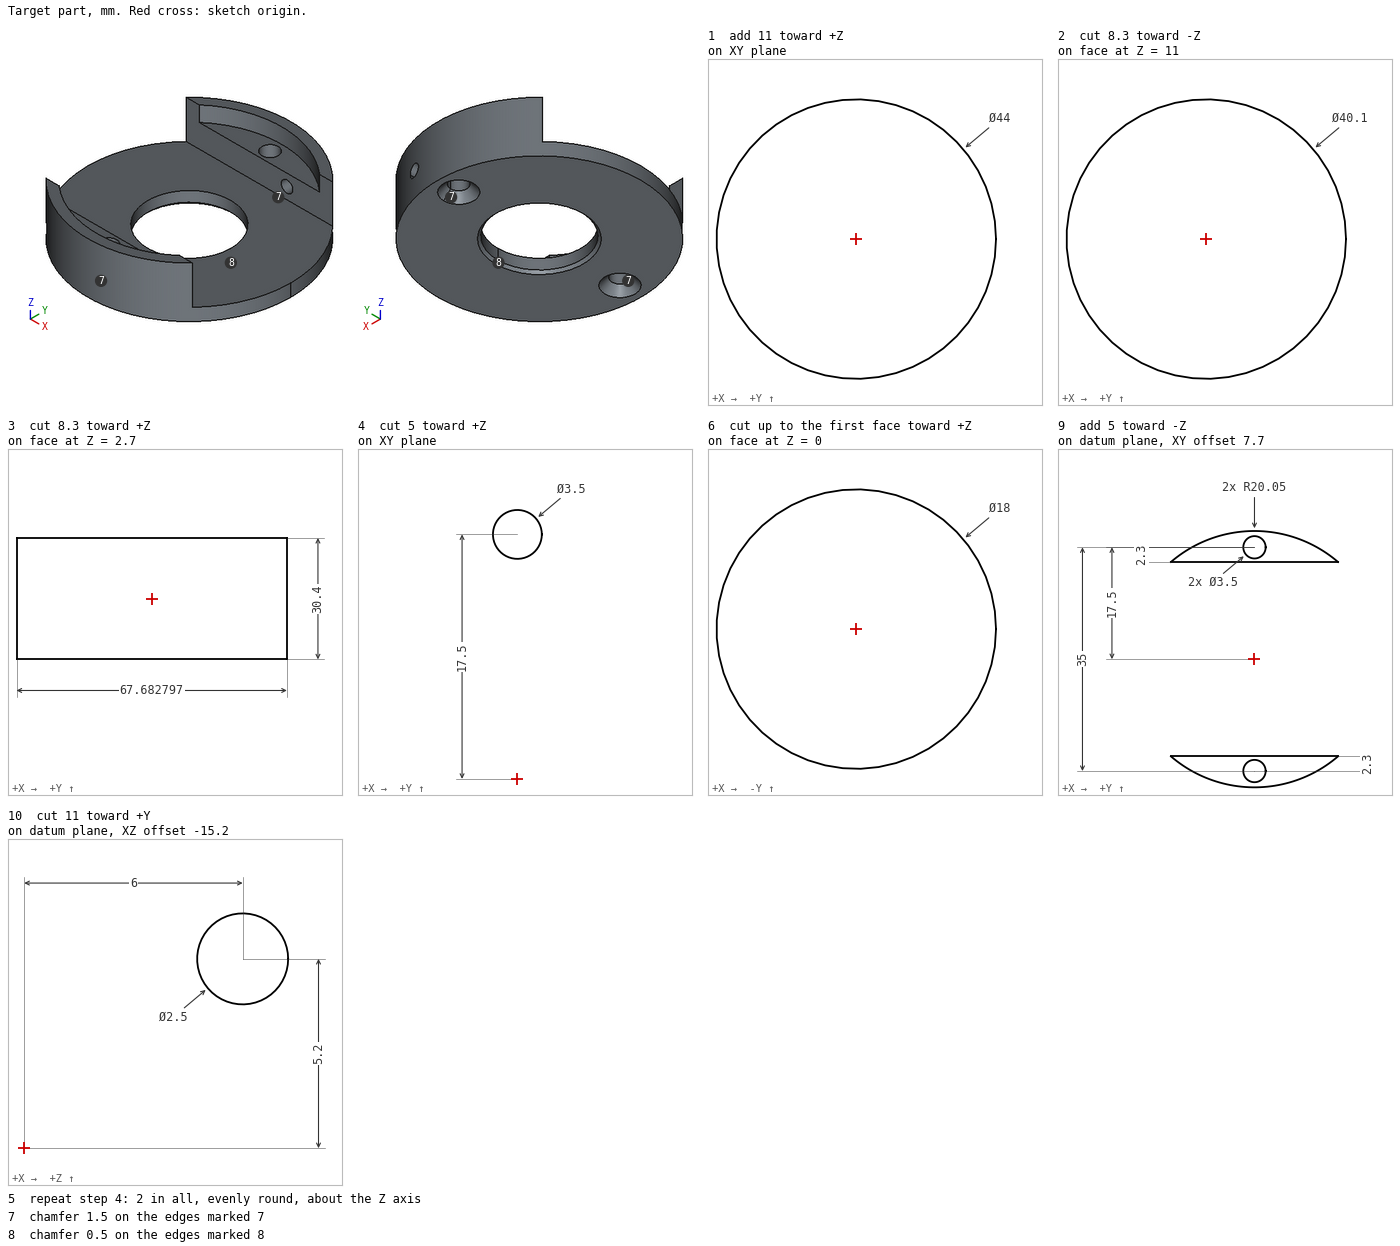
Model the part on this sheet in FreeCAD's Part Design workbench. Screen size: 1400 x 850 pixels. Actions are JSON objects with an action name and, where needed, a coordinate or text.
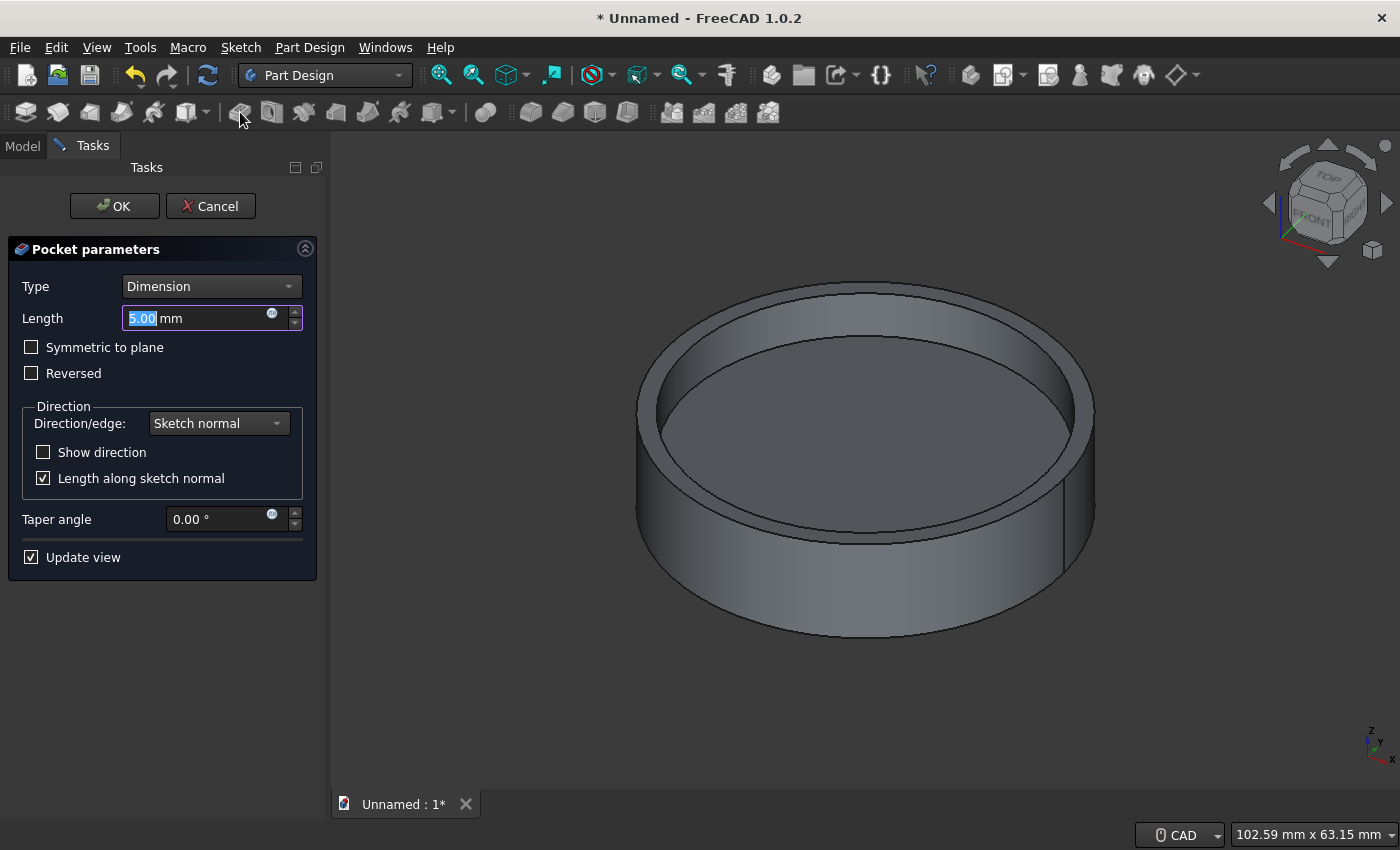
{"action": "type", "text": "8.3"}
{"action": "key", "text": "Tab"}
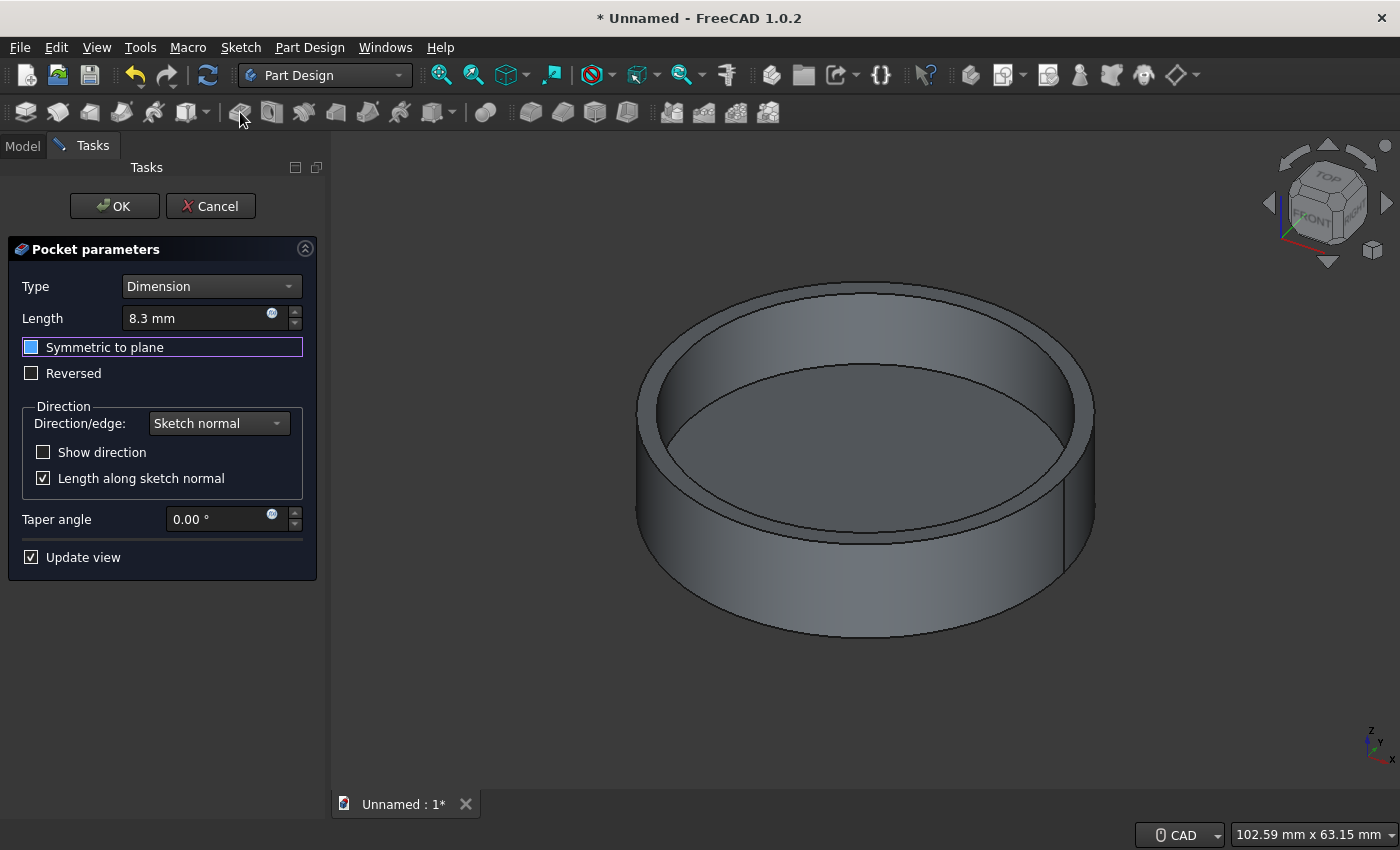
{"action": "left_click", "coordinate": [115, 206]}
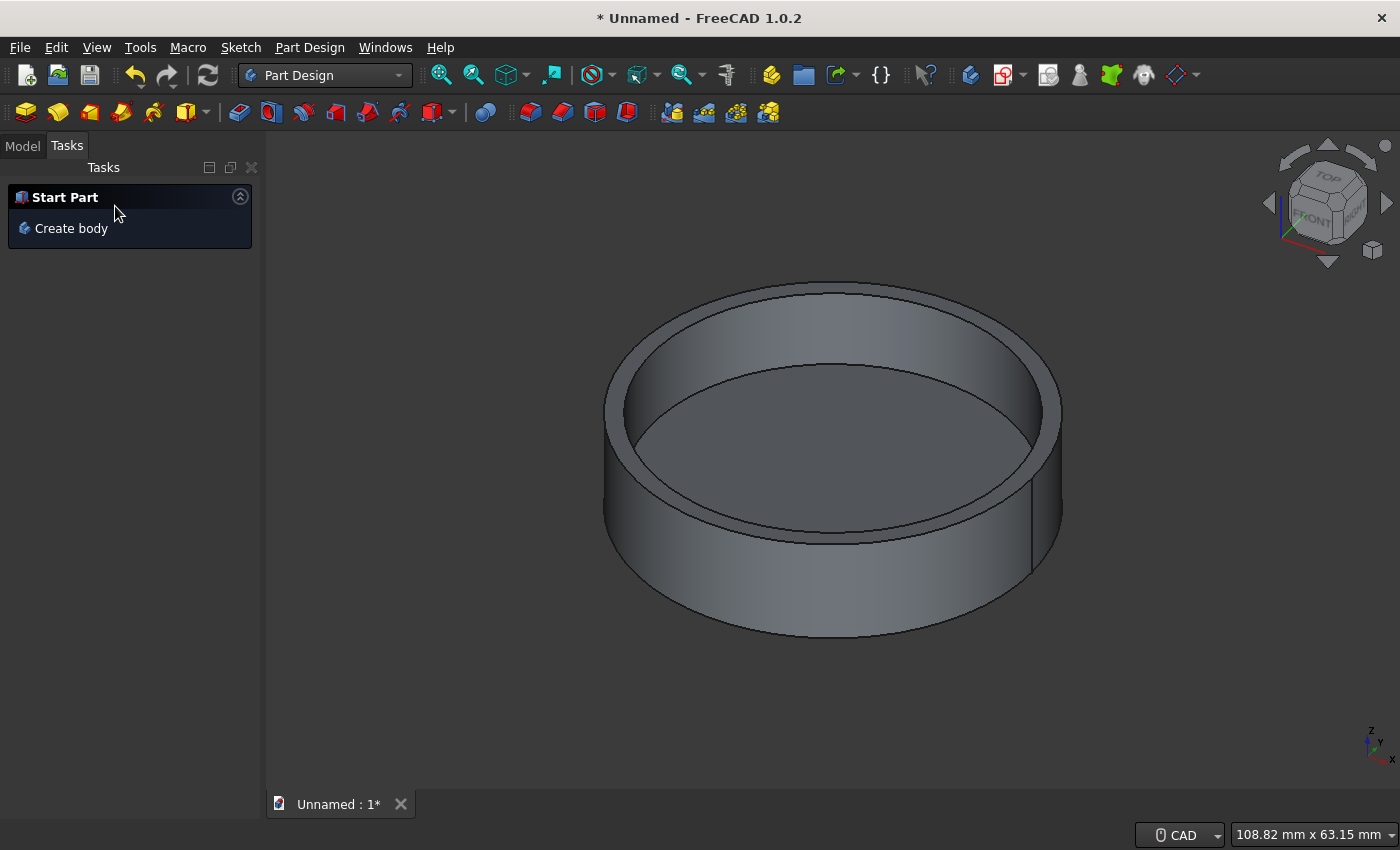
{"action": "left_click", "coordinate": [833, 483]}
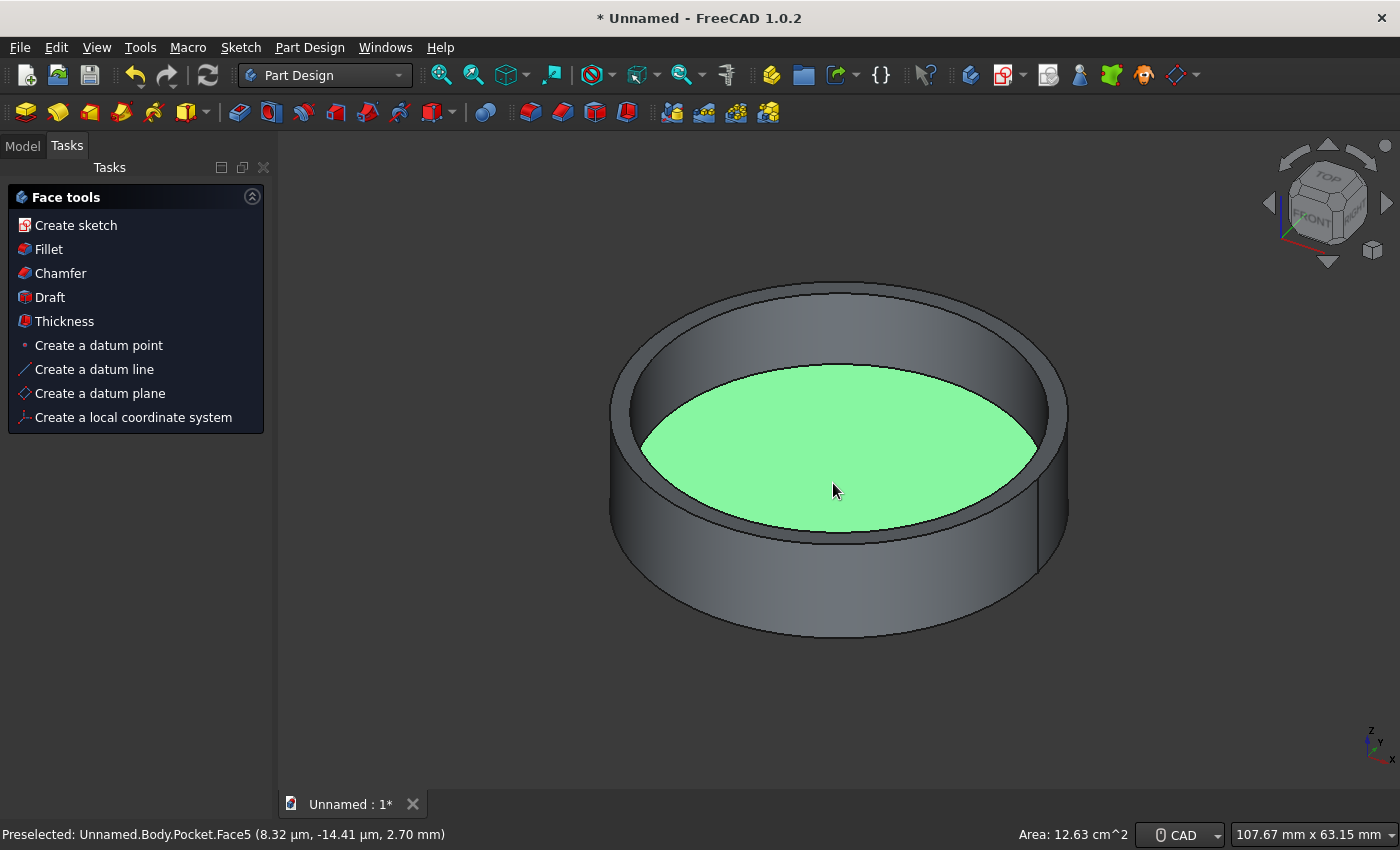
{"action": "left_click", "coordinate": [1004, 76]}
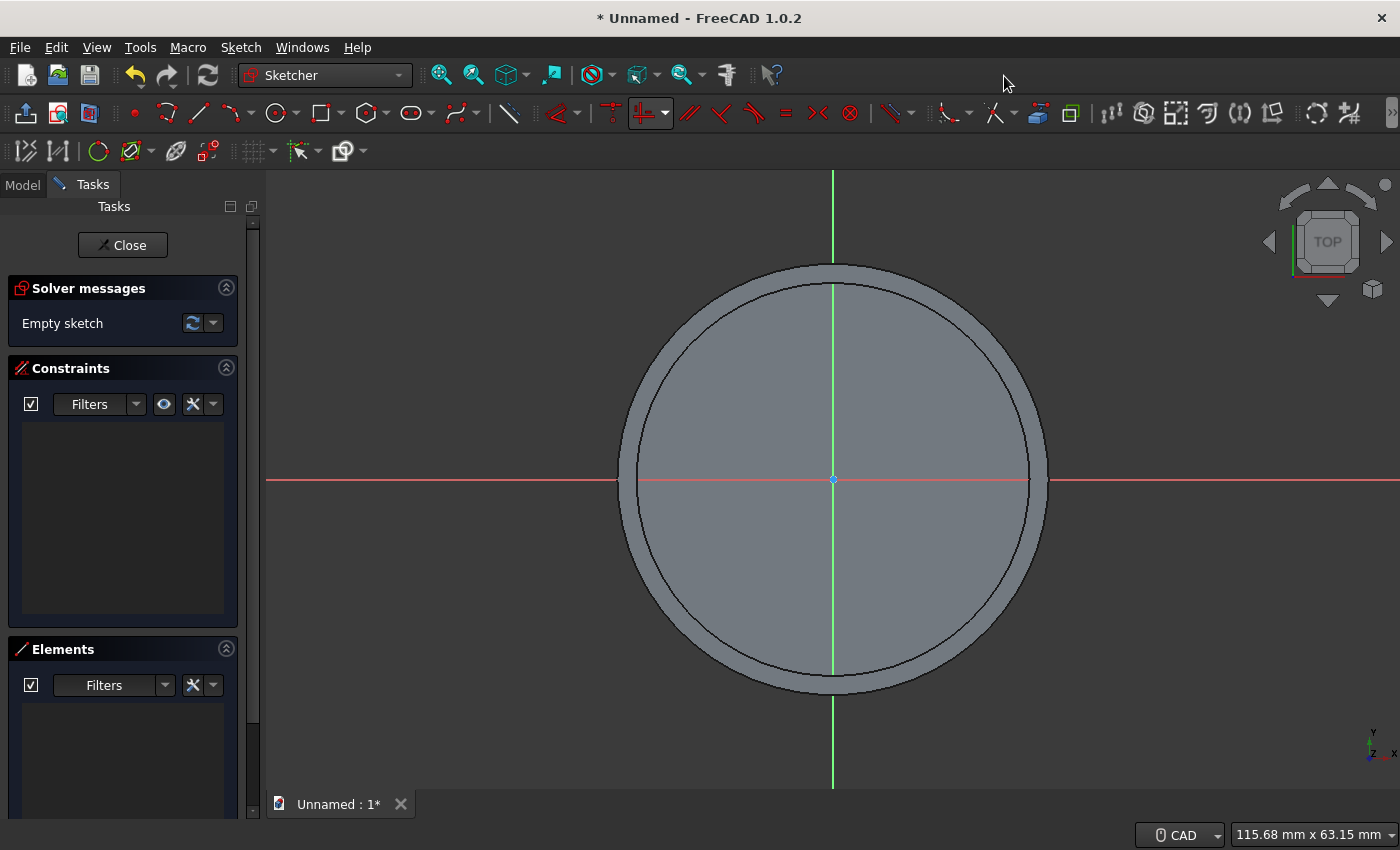
{"action": "left_click", "coordinate": [90, 114]}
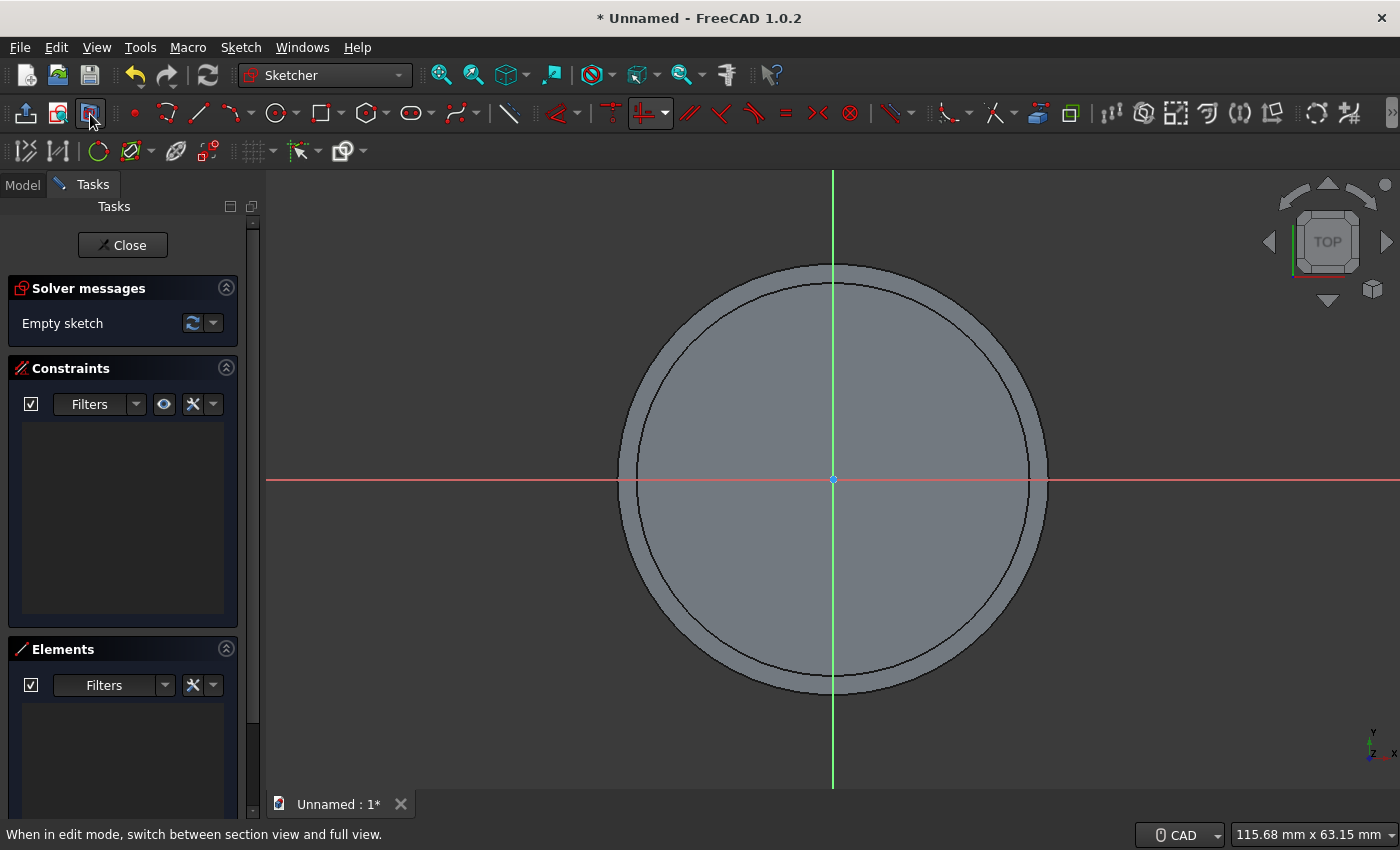
{"action": "left_click", "coordinate": [344, 114]}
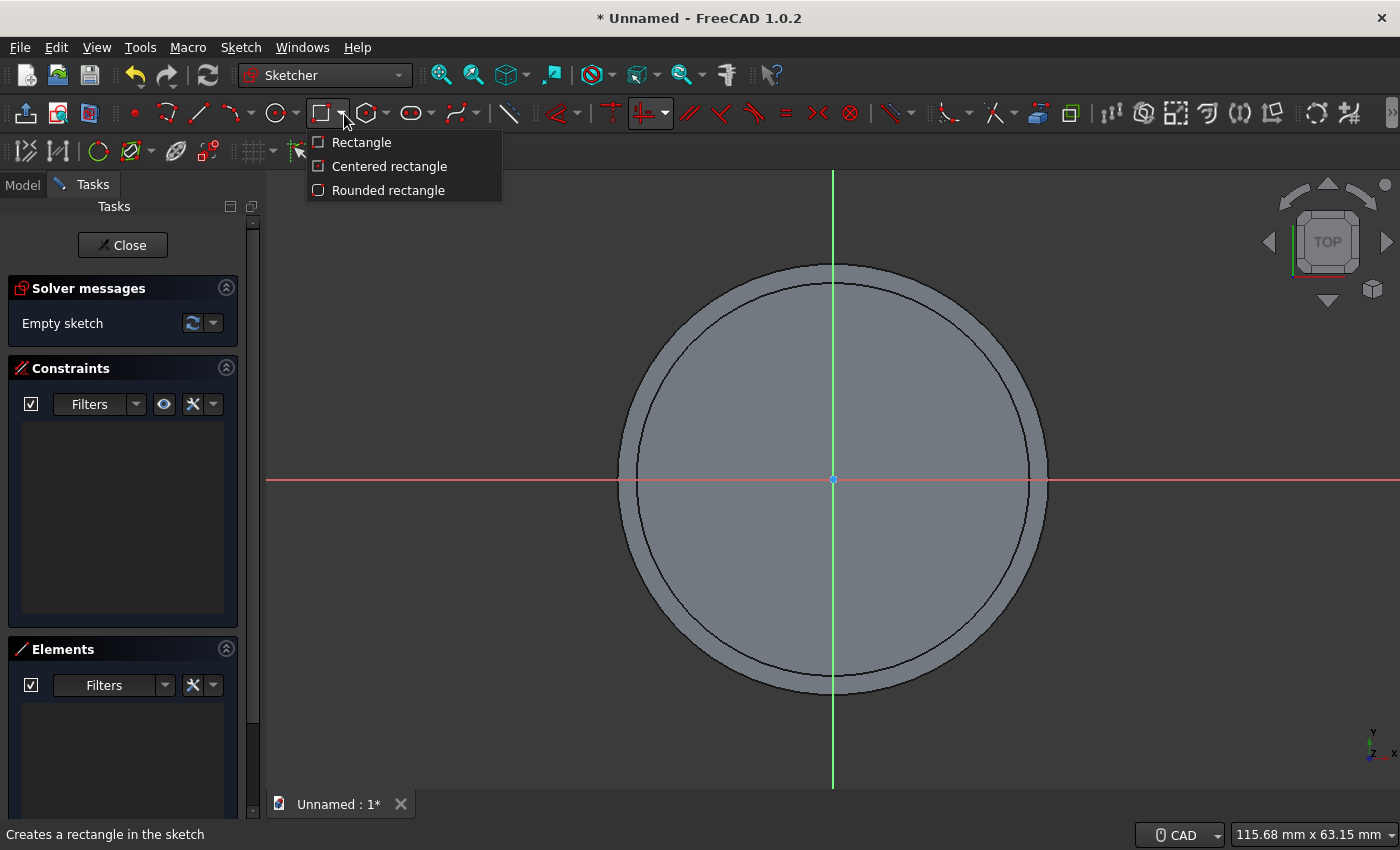
{"action": "left_click", "coordinate": [404, 166]}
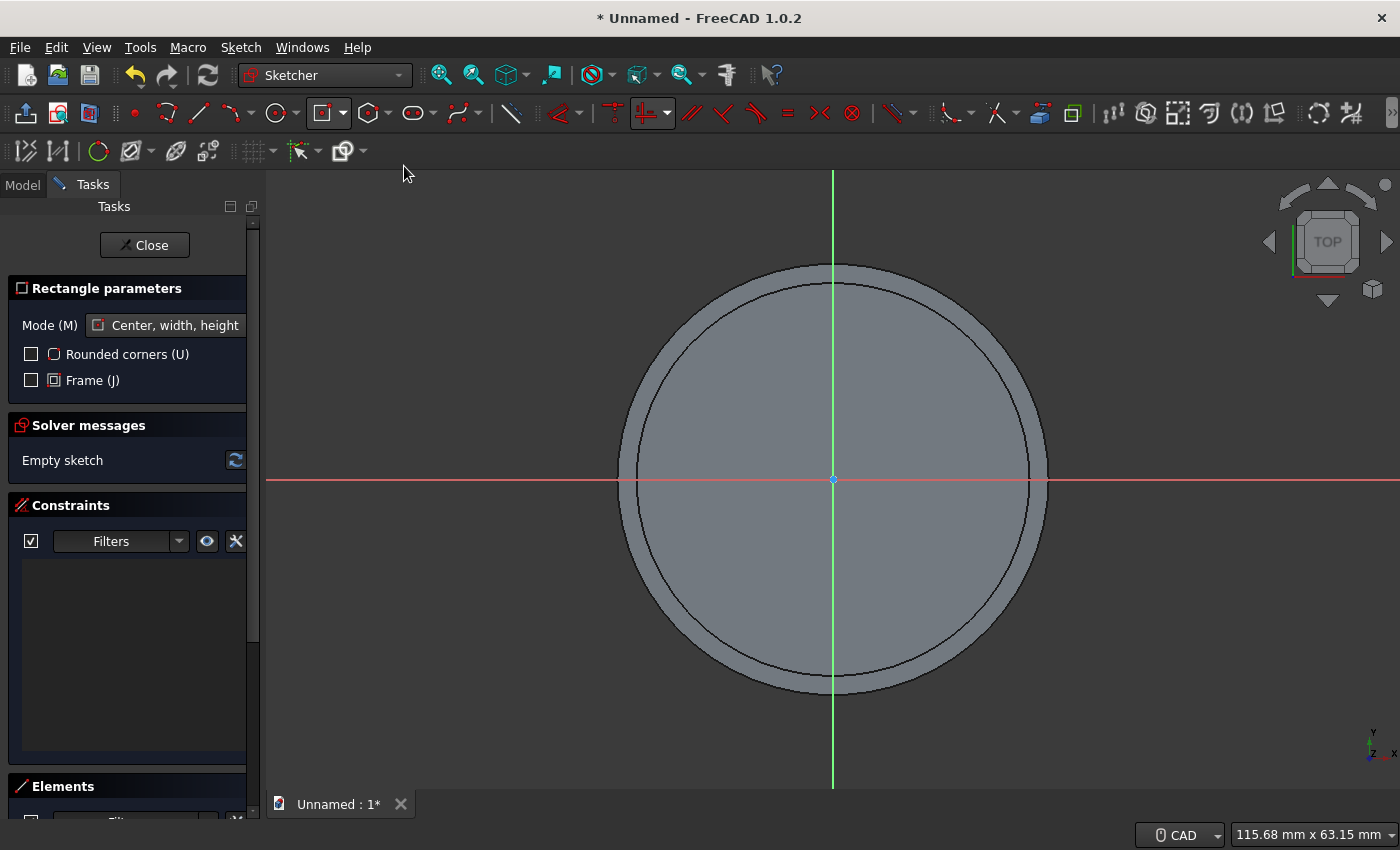
{"action": "left_click", "coordinate": [833, 480]}
{"action": "left_click", "coordinate": [1165, 330]}
{"action": "key", "text": "Escape"}